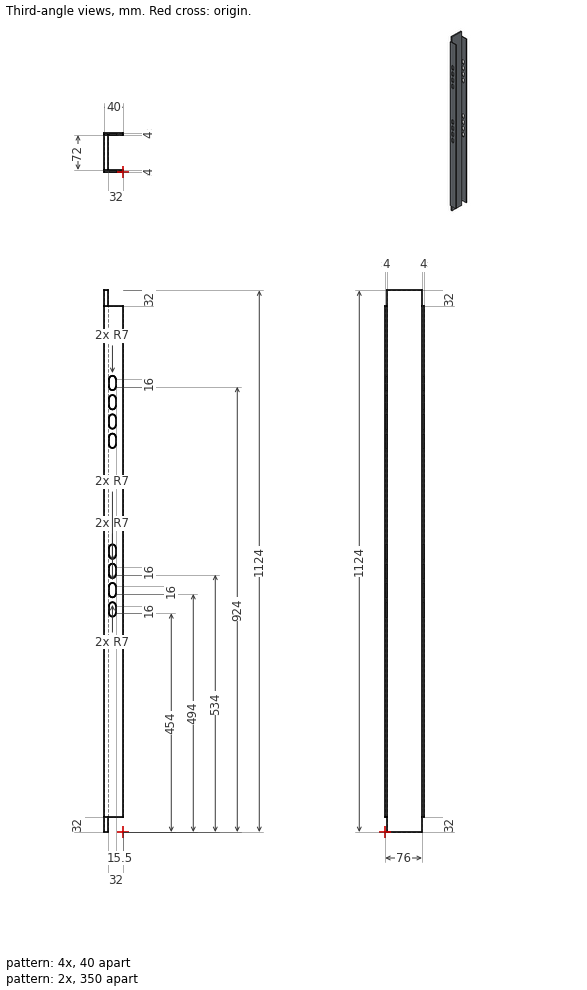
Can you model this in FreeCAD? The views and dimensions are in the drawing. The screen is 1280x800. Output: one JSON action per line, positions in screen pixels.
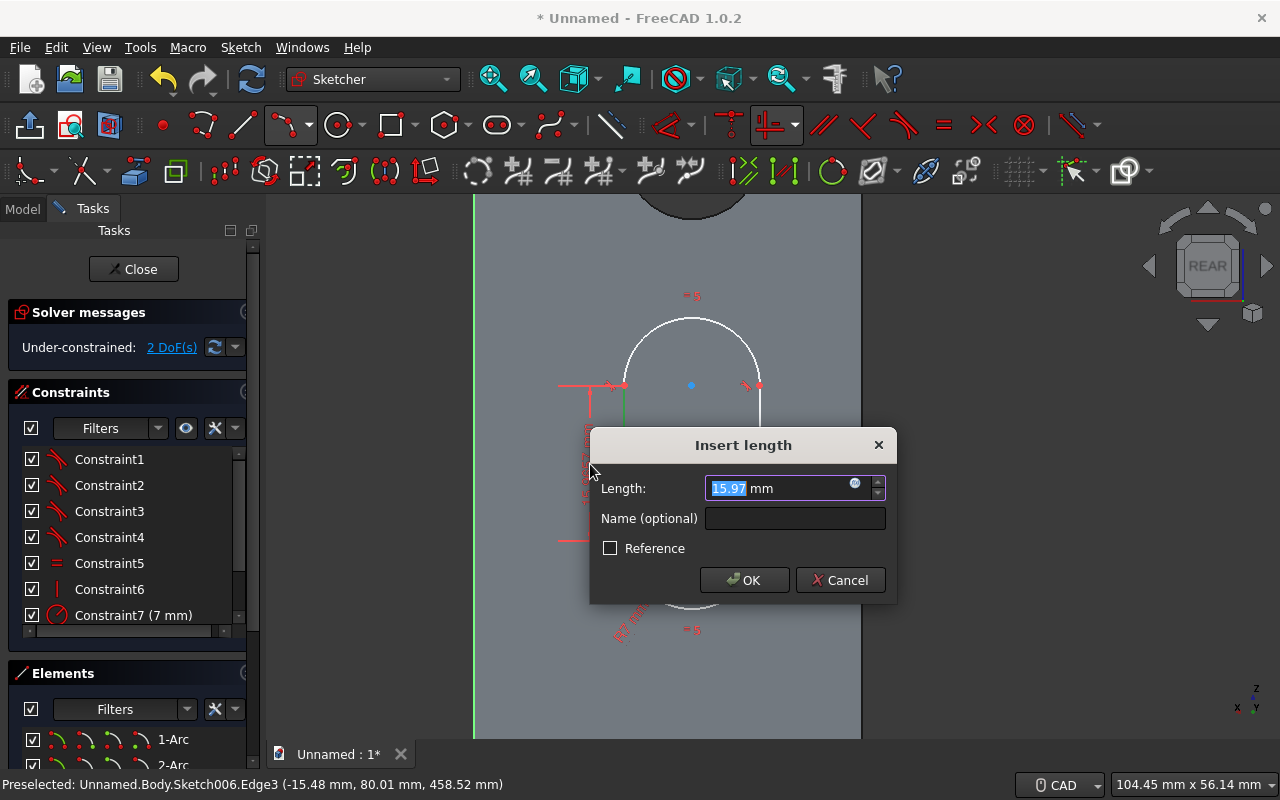
{"action": "type", "text": "16"}
{"action": "key", "text": "Return"}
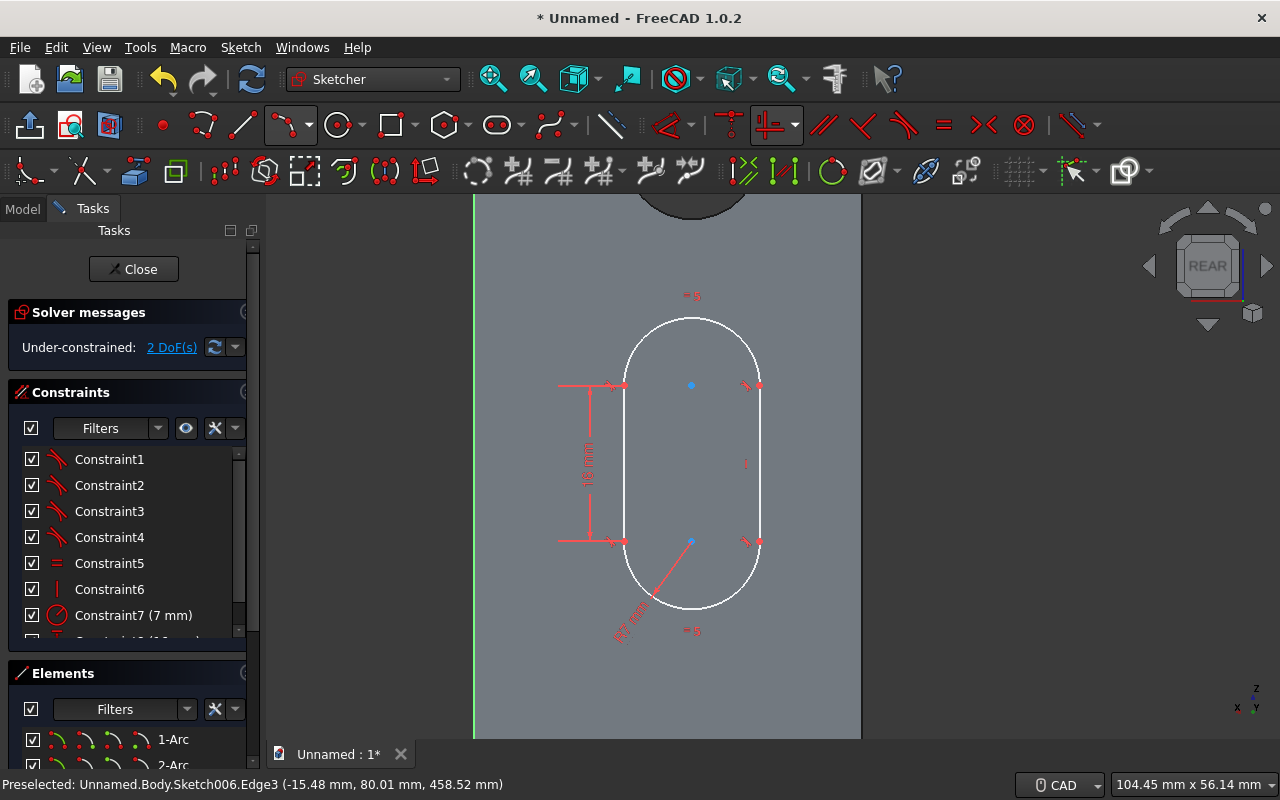
{"action": "left_click", "coordinate": [624, 541]}
{"action": "left_click", "coordinate": [440, 626]}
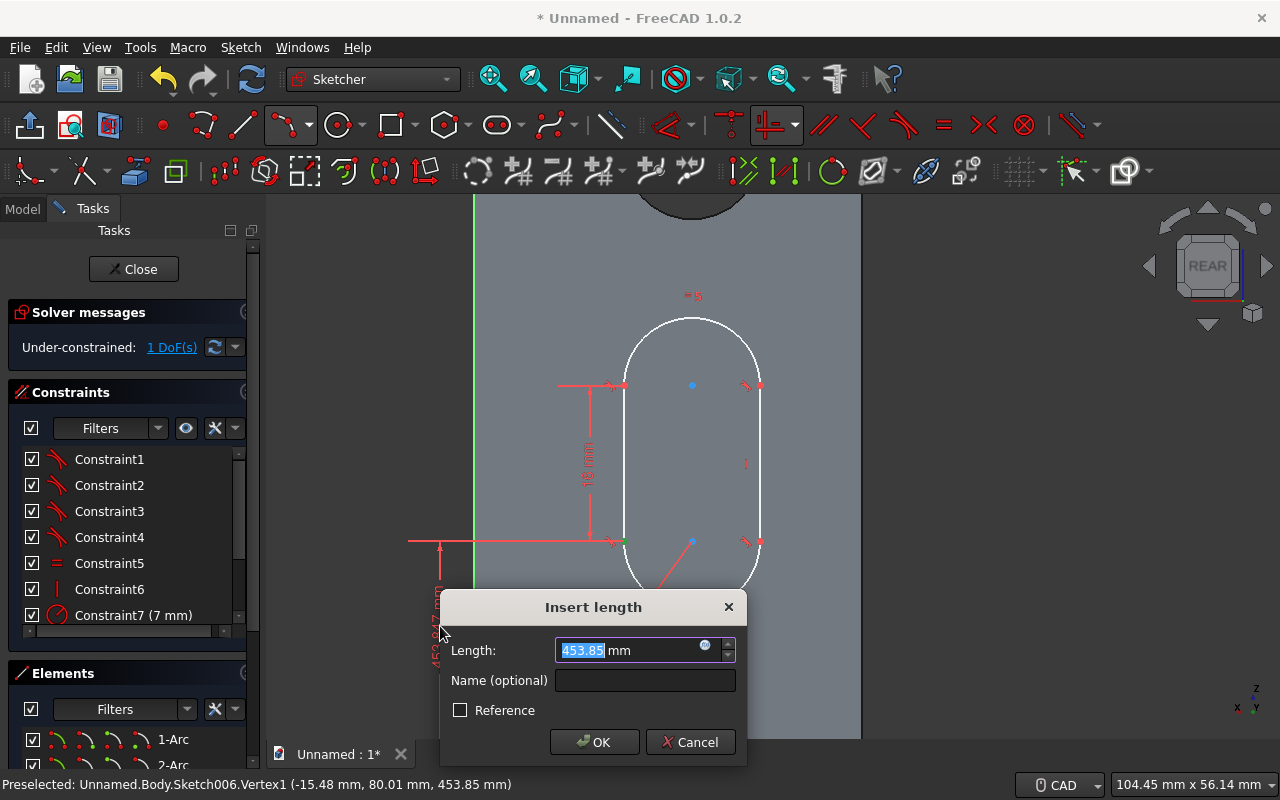
{"action": "type", "text": "454"}
{"action": "key", "text": "Return"}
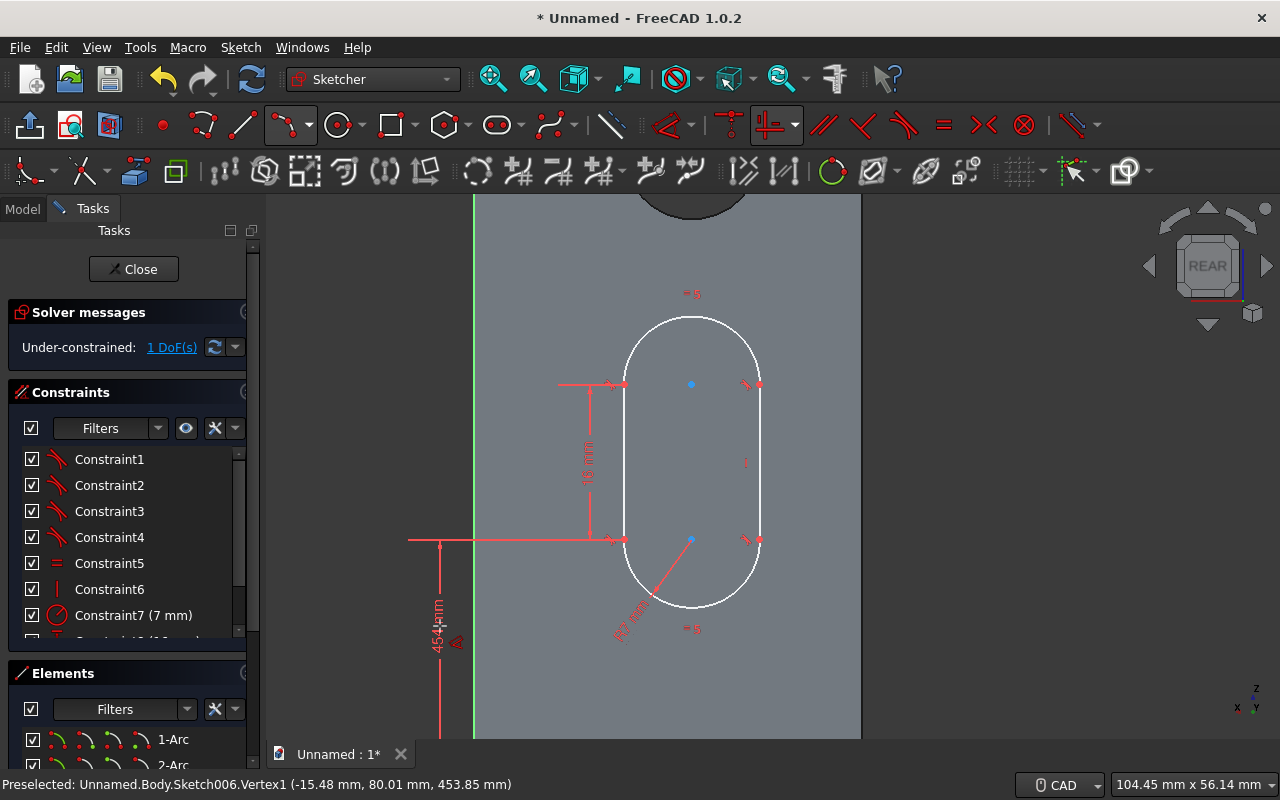
{"action": "left_click", "coordinate": [624, 540]}
{"action": "left_click", "coordinate": [549, 506]}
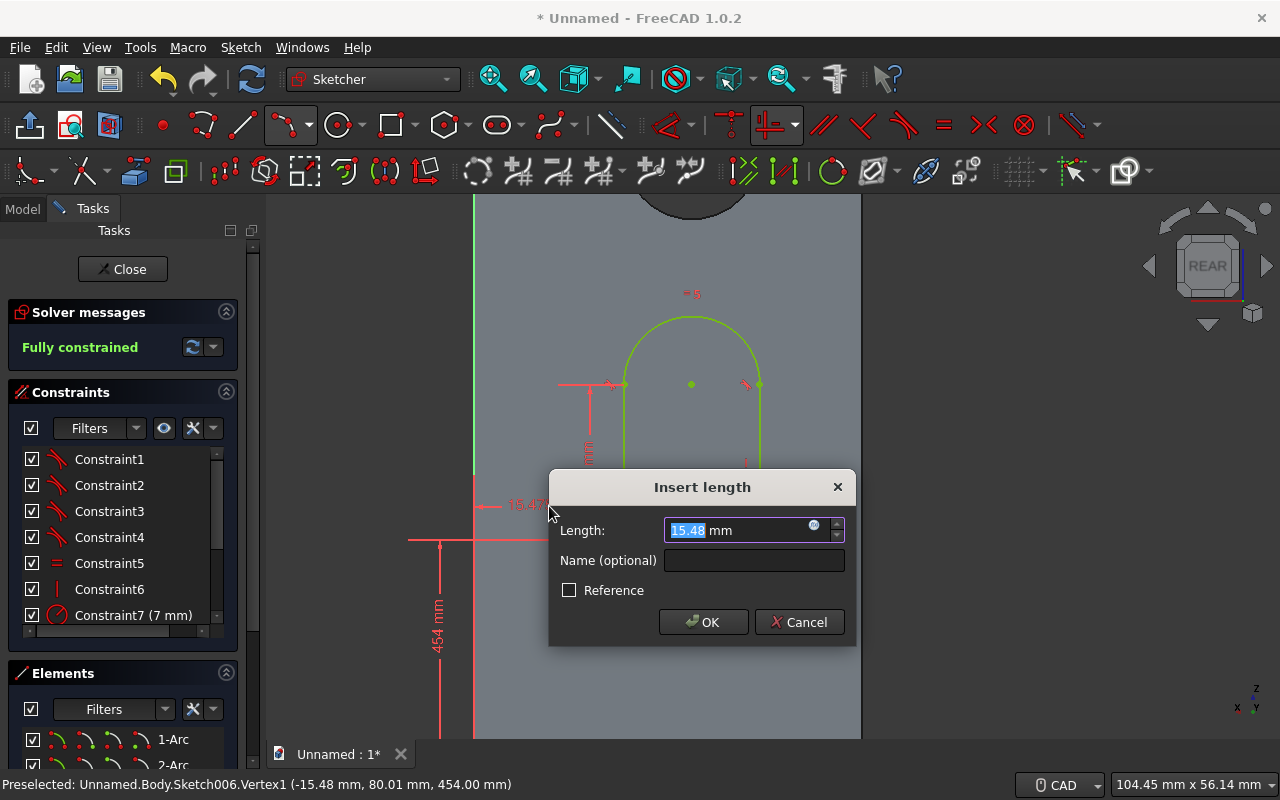
{"action": "type", "text": "15.5"}
{"action": "key", "text": "Return"}
{"action": "key", "text": "Escape"}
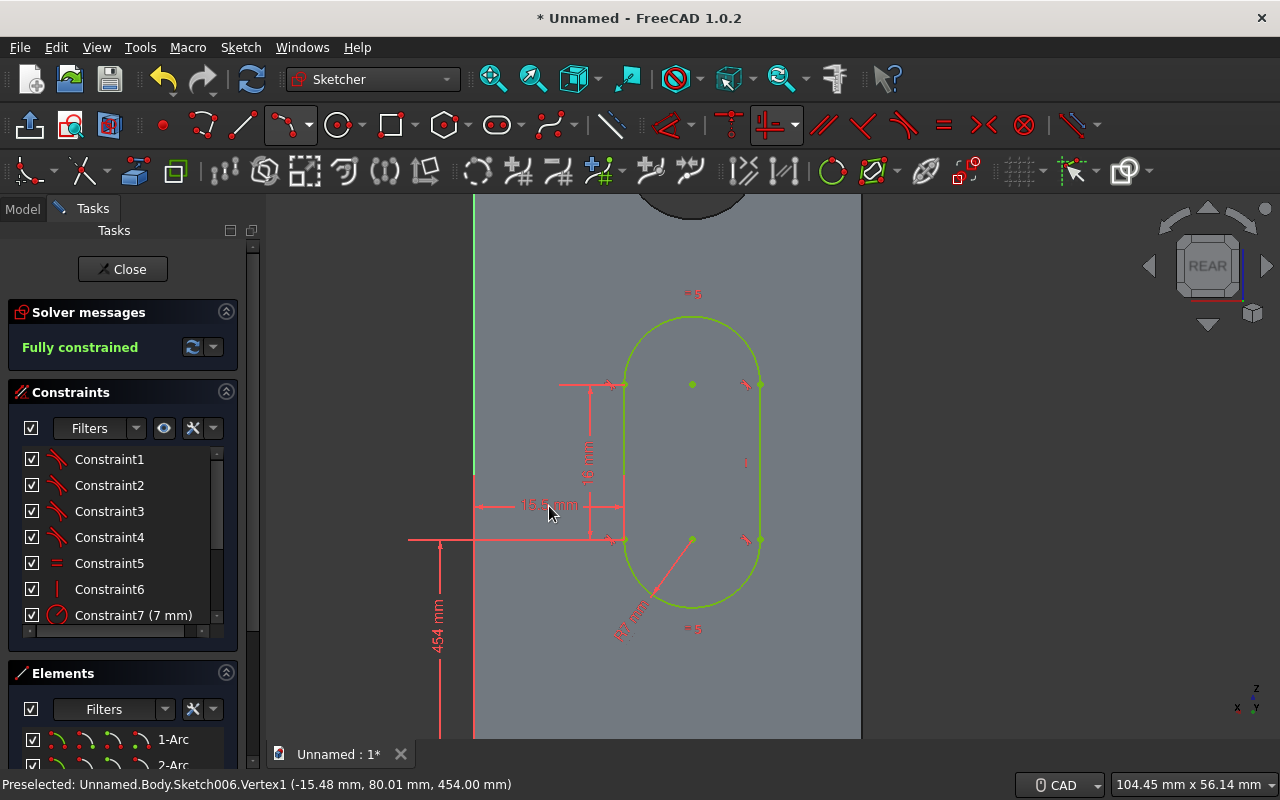
{"action": "left_click", "coordinate": [123, 269]}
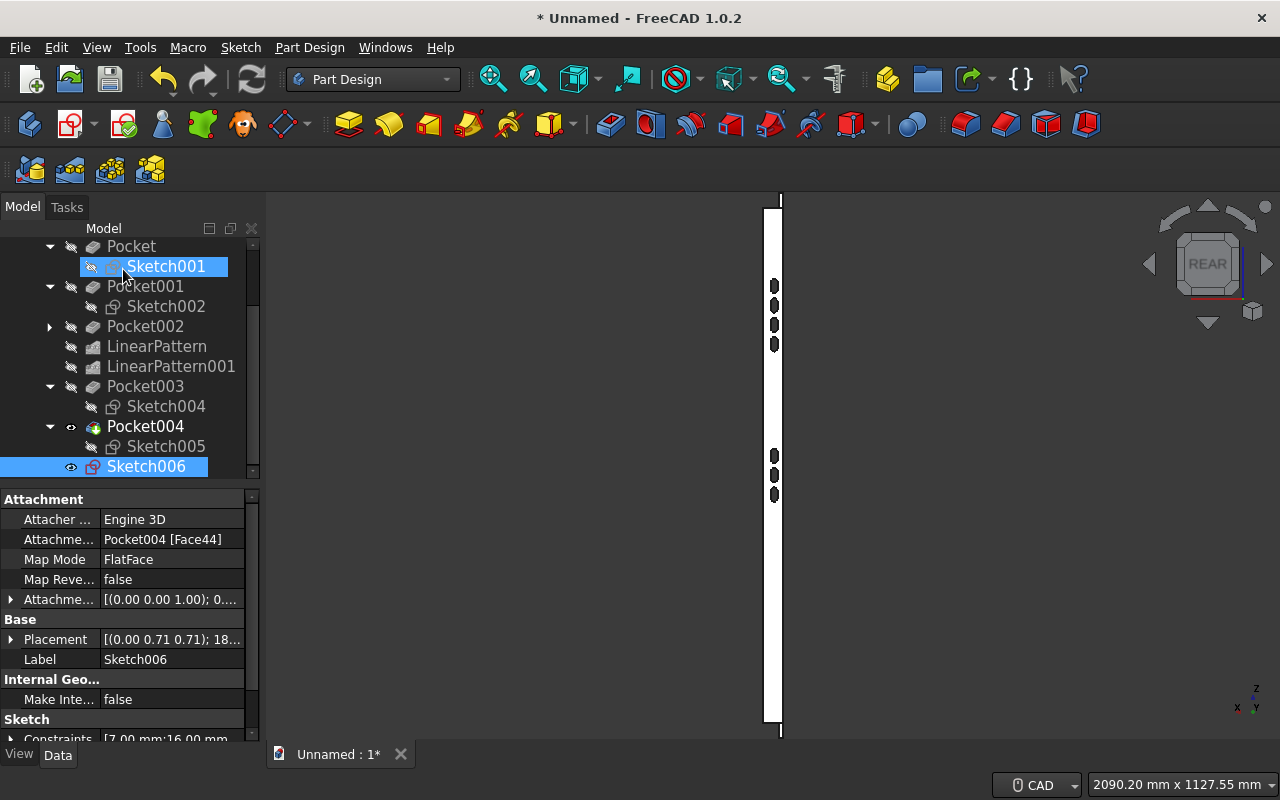
{"action": "left_click", "coordinate": [612, 124]}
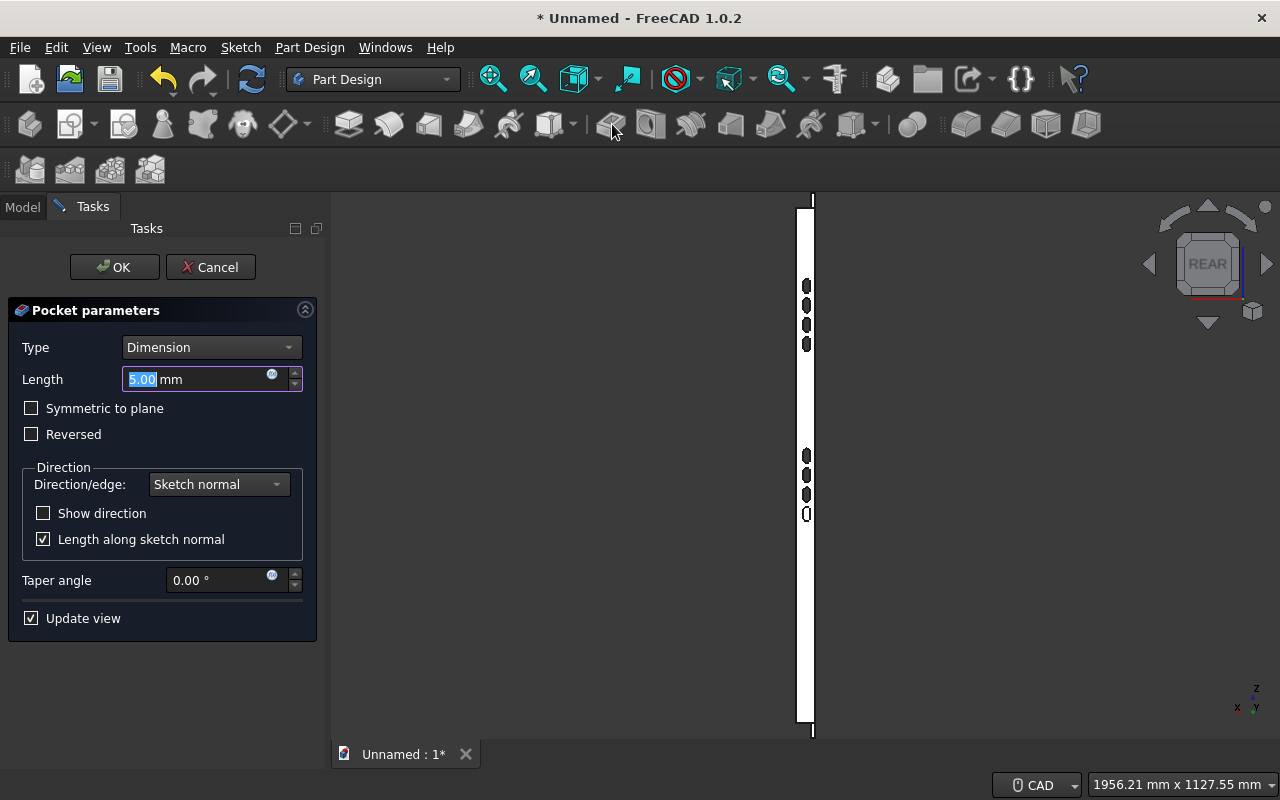
{"action": "left_click", "coordinate": [212, 348]}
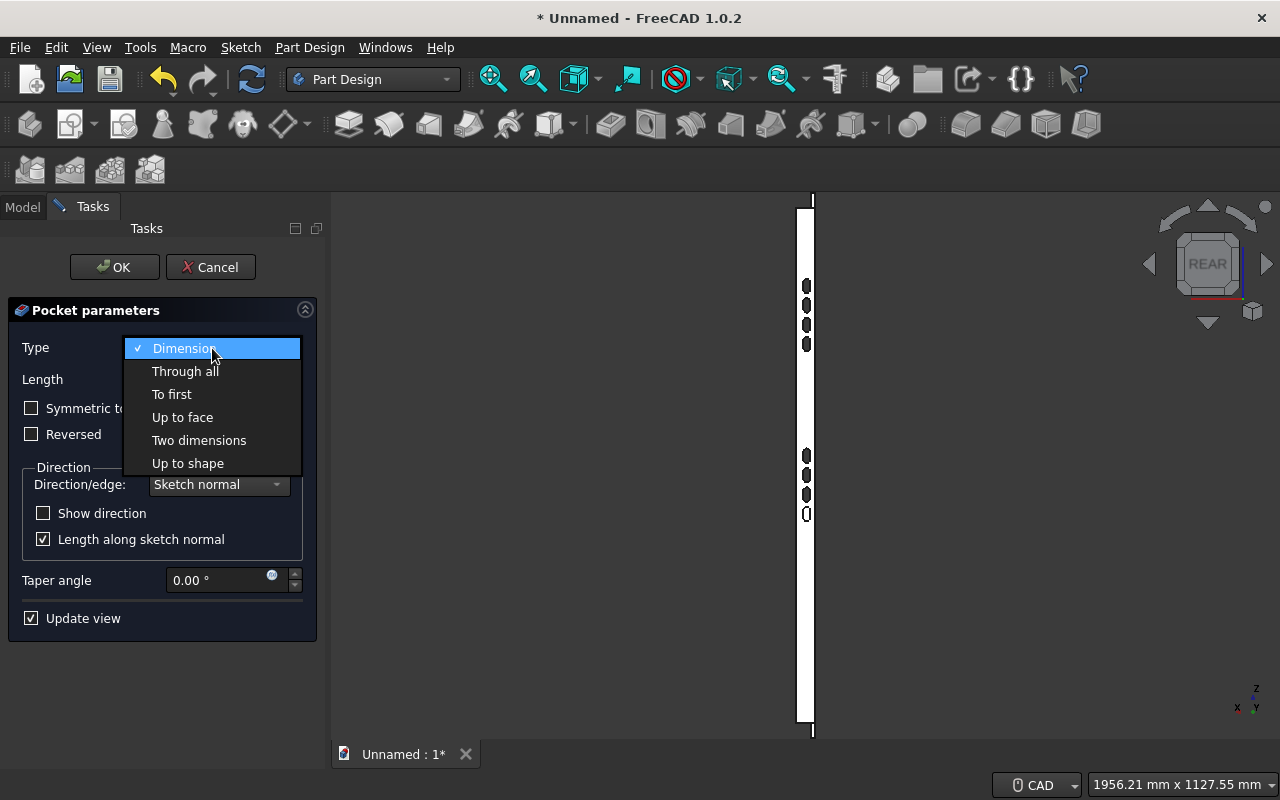
{"action": "left_click", "coordinate": [212, 372]}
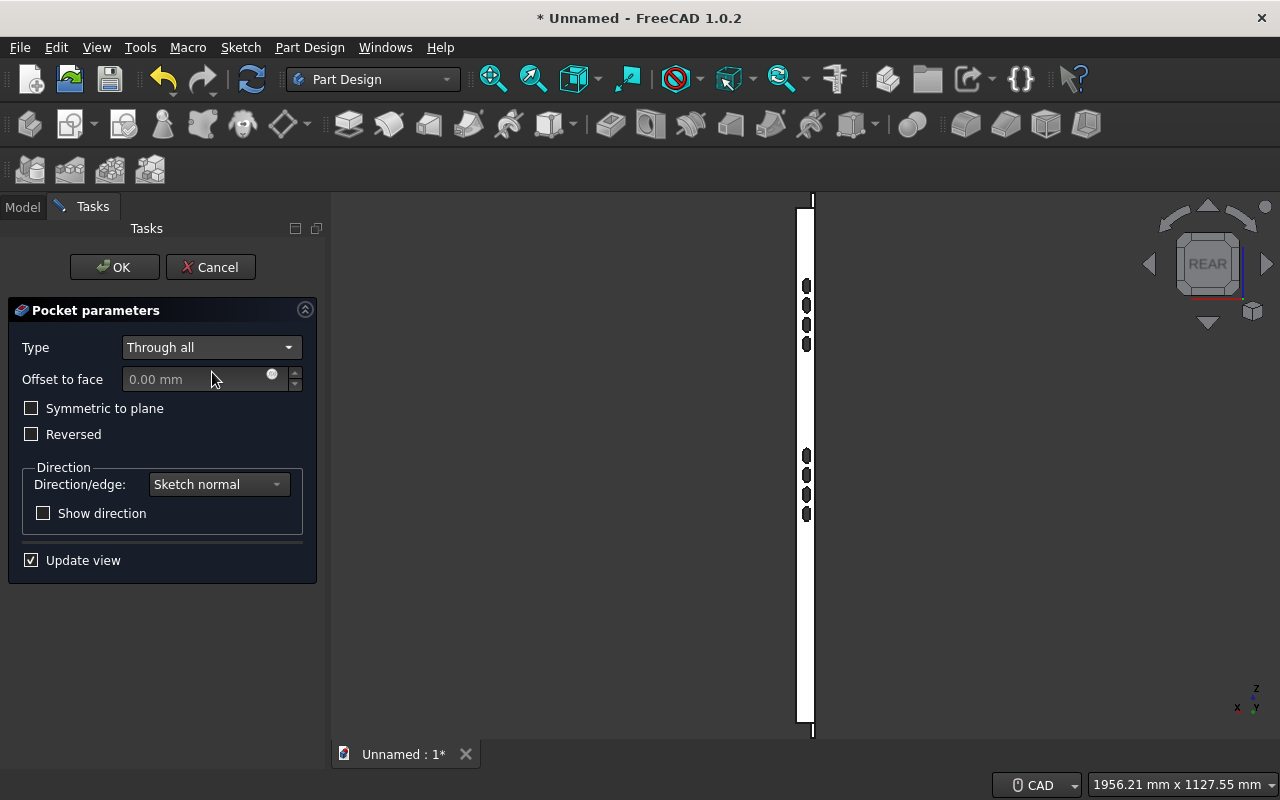
{"action": "left_click", "coordinate": [115, 267]}